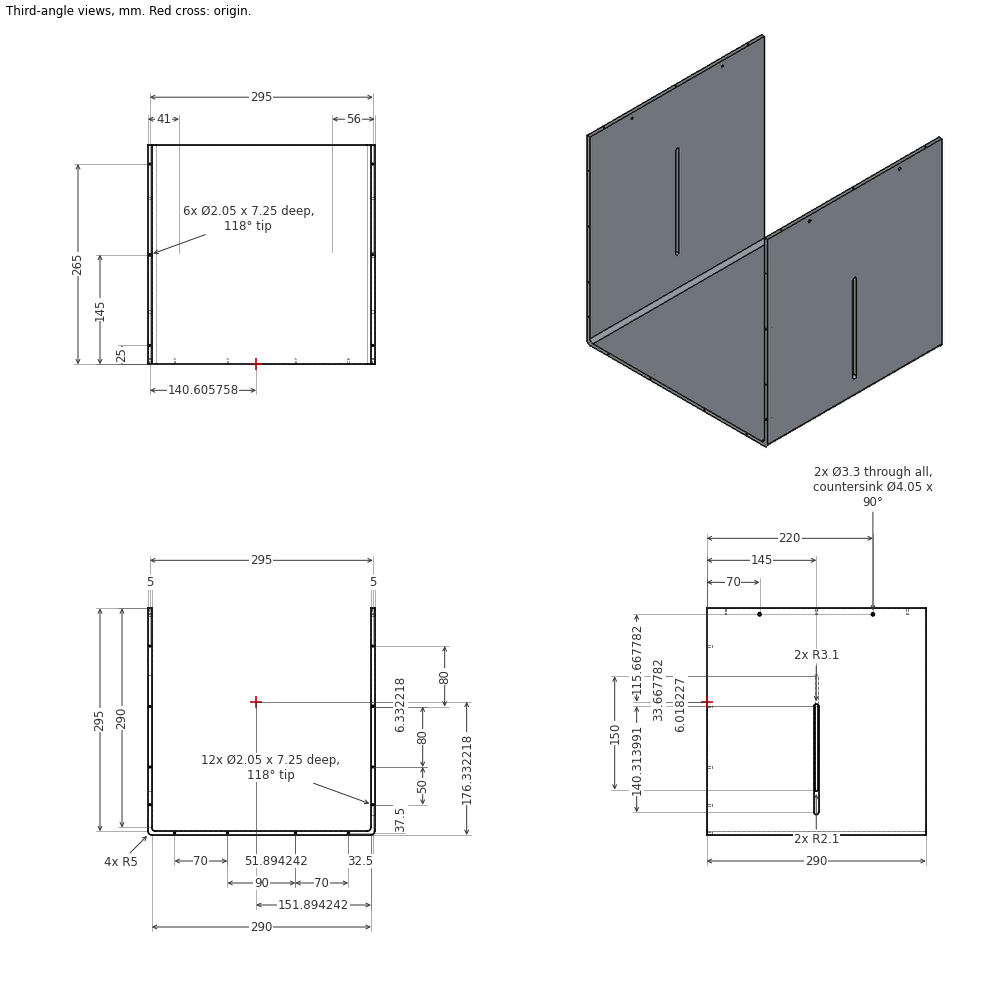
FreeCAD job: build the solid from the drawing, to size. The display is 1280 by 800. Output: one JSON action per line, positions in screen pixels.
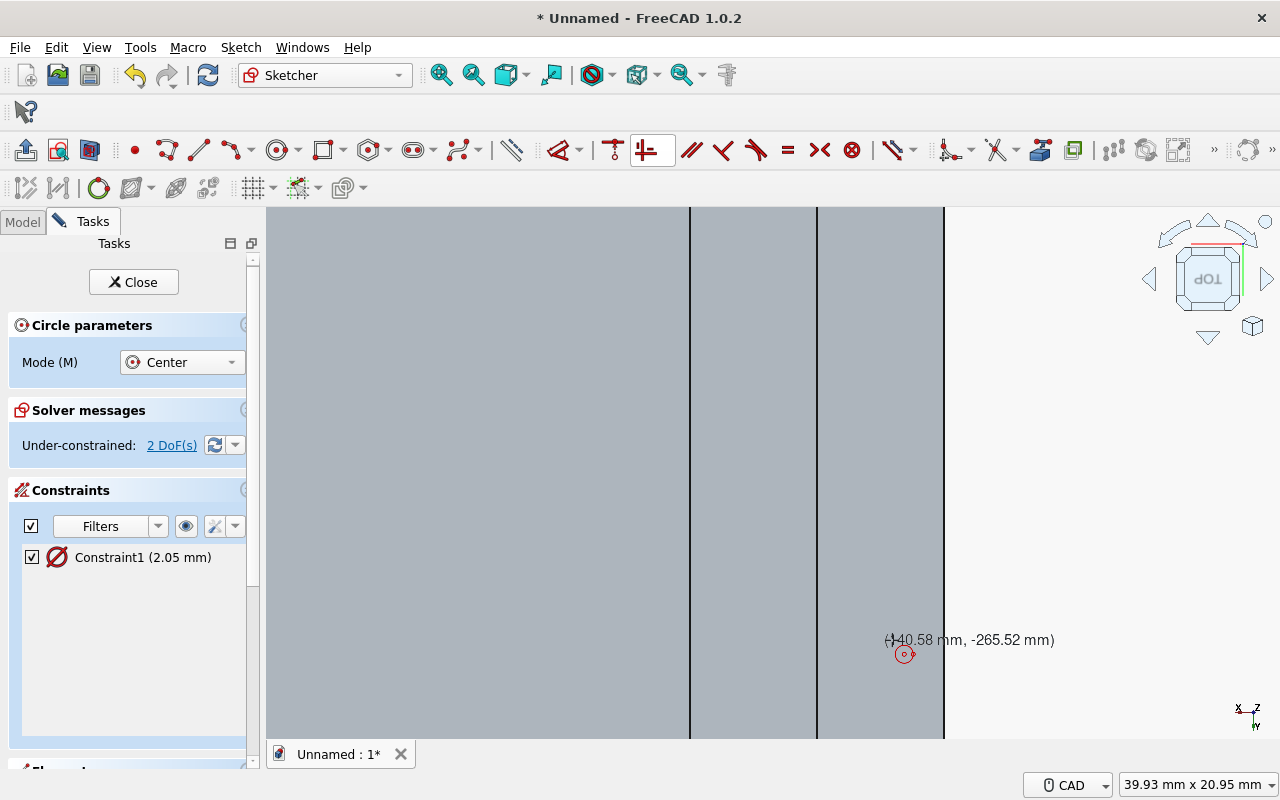
{"action": "scroll", "coordinate": [892, 640], "scroll_direction": "down", "scroll_amount": 15}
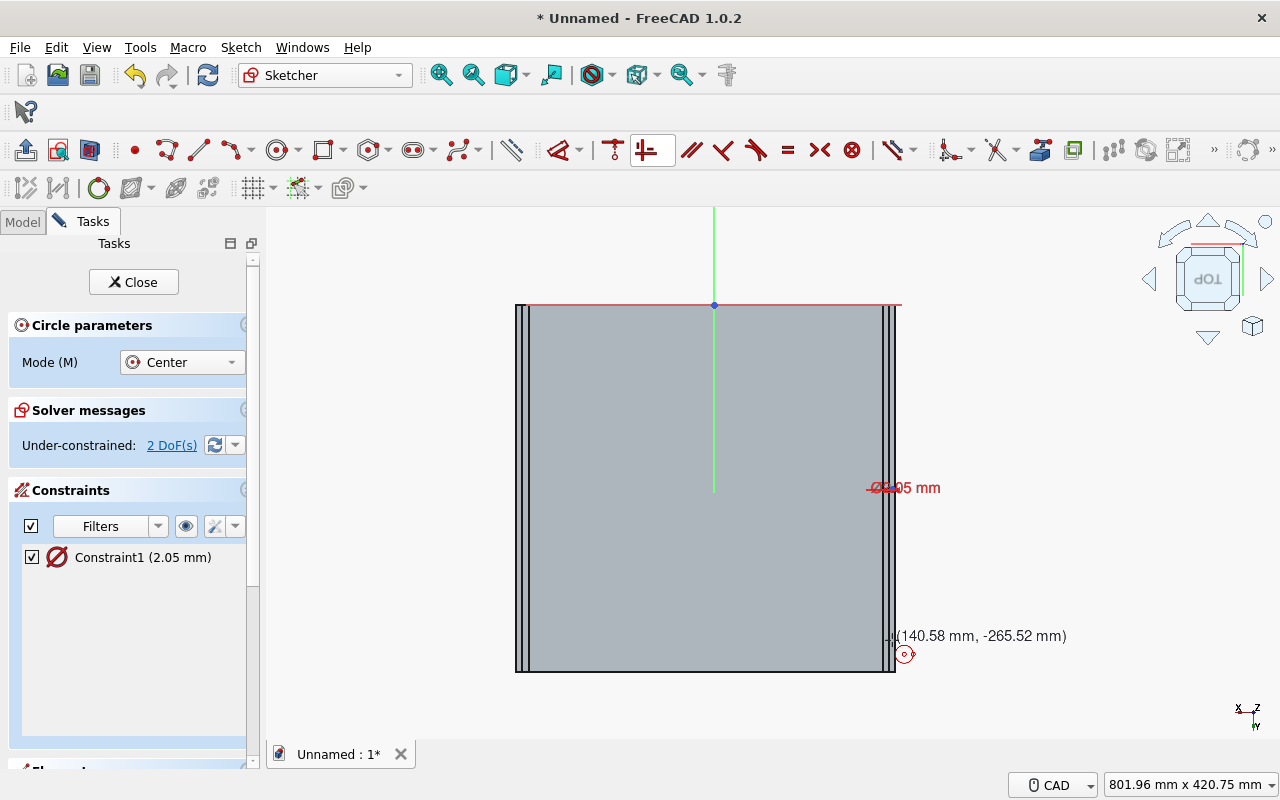
{"action": "left_click", "coordinate": [892, 640]}
{"action": "mouse_move", "coordinate": [893, 639]}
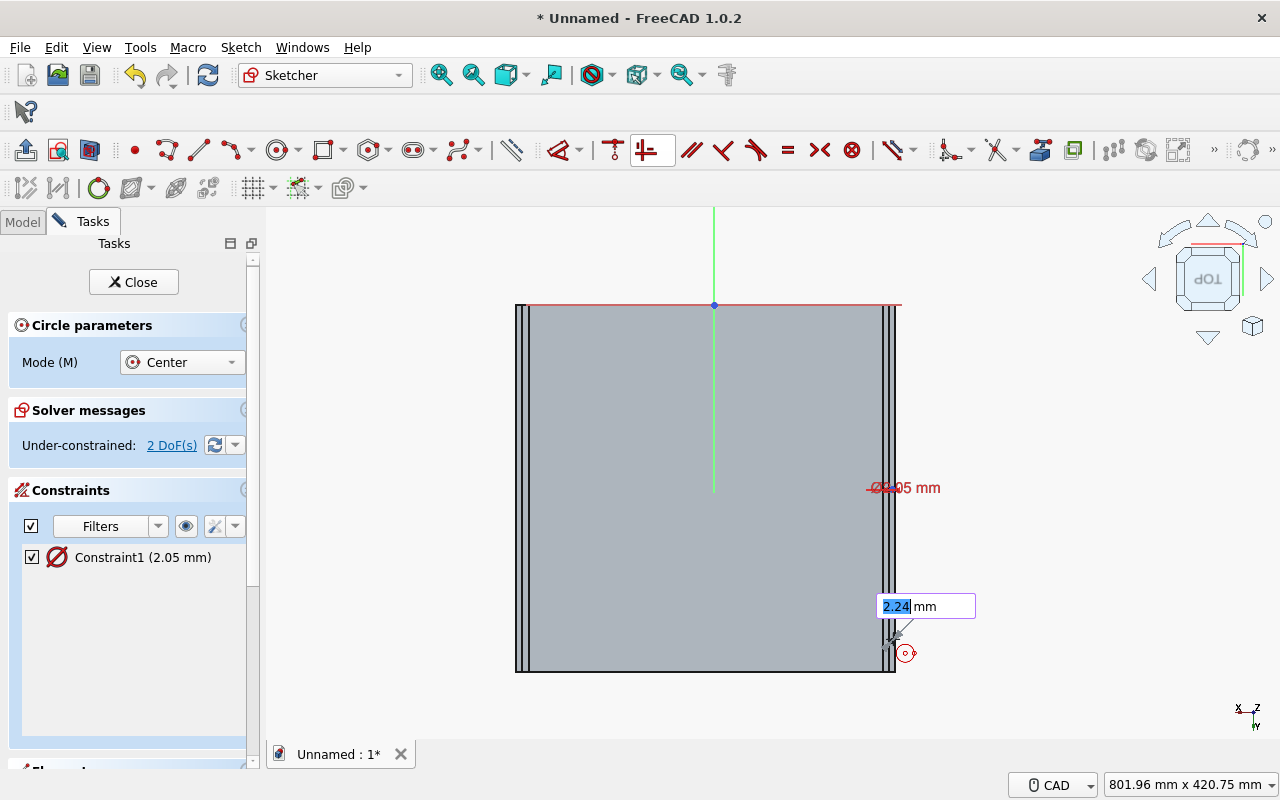
{"action": "type", "text": "2.05"}
{"action": "key", "text": "Return"}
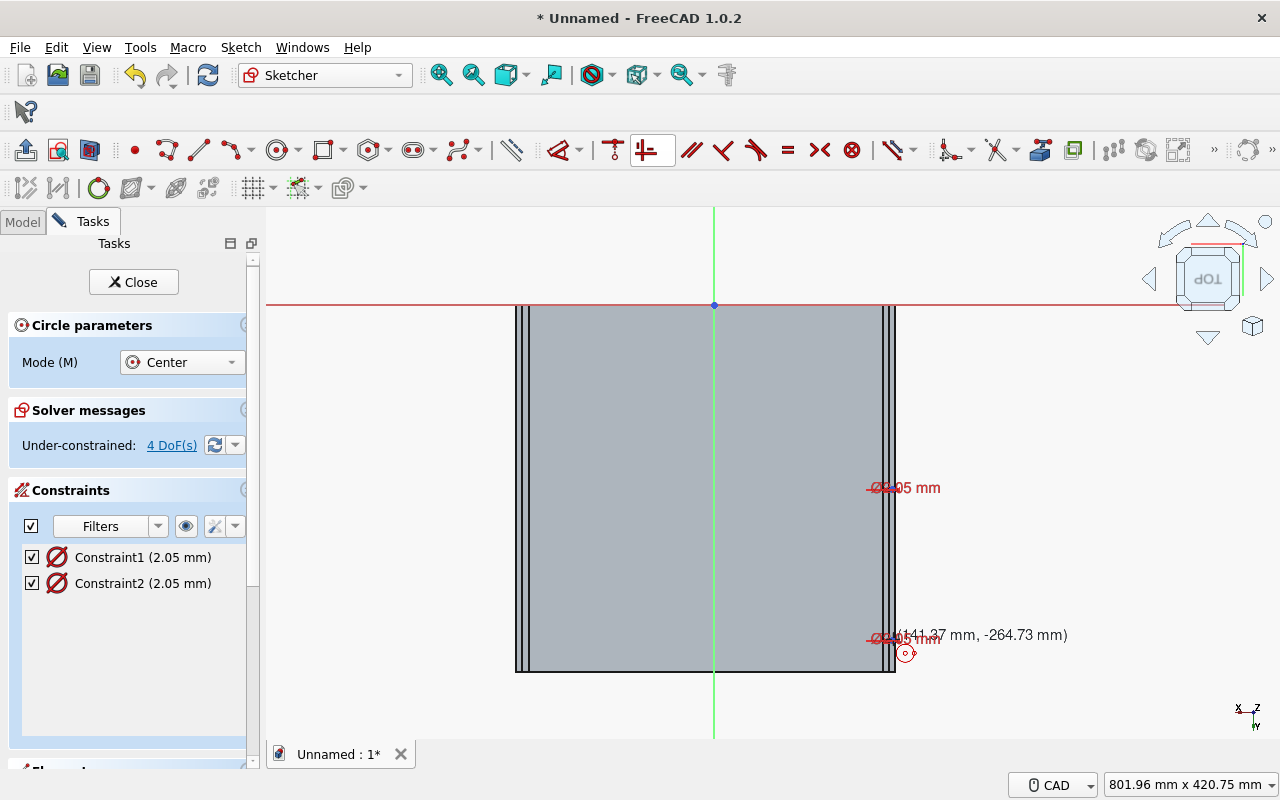
{"action": "scroll", "coordinate": [892, 337], "scroll_direction": "up", "scroll_amount": 15}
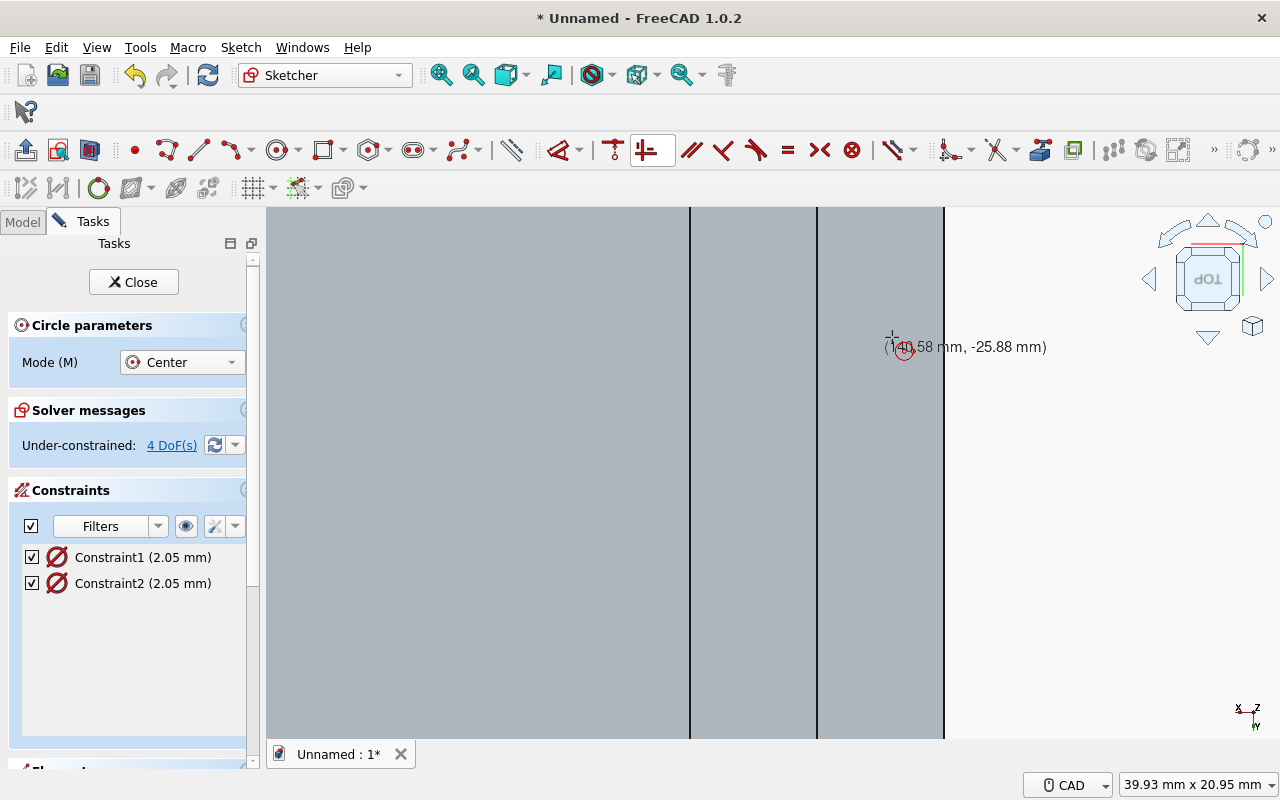
{"action": "scroll", "coordinate": [892, 337], "scroll_direction": "down", "scroll_amount": 15}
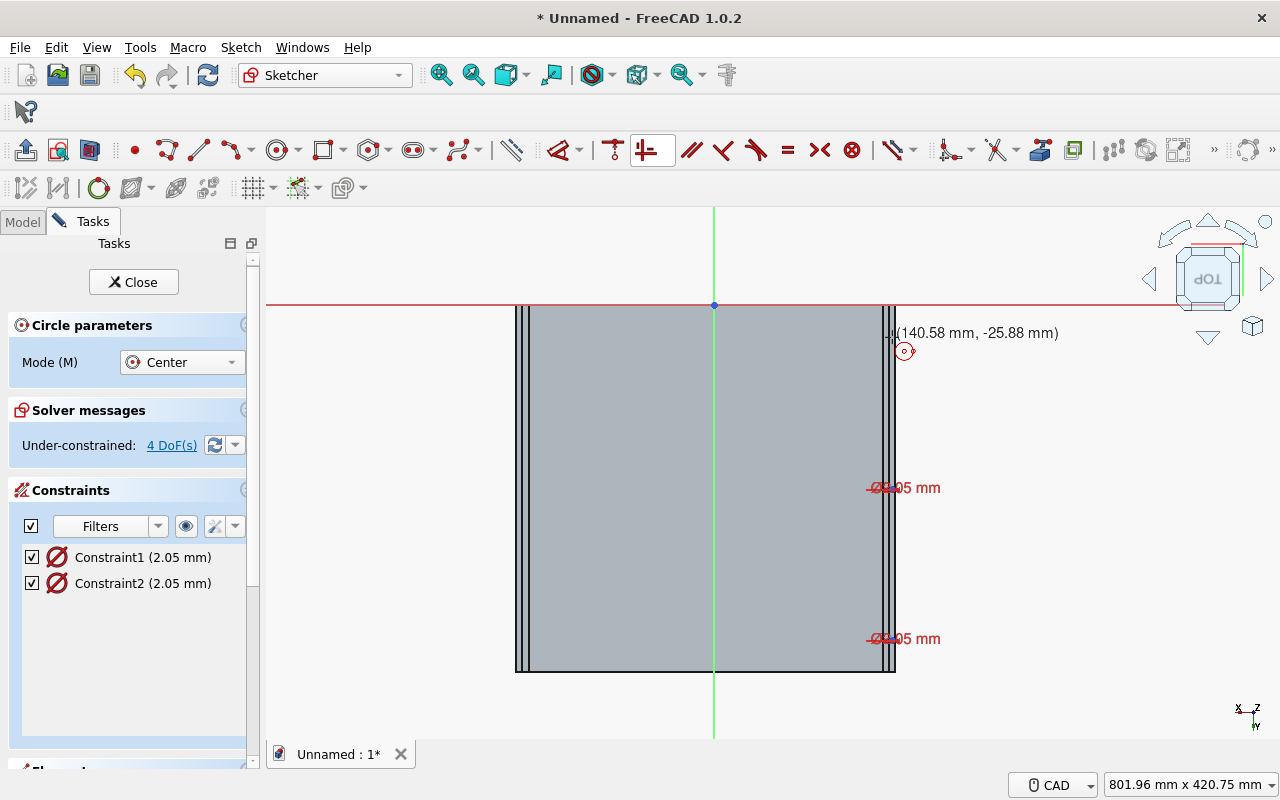
{"action": "left_click", "coordinate": [892, 337]}
{"action": "mouse_move", "coordinate": [893, 336]}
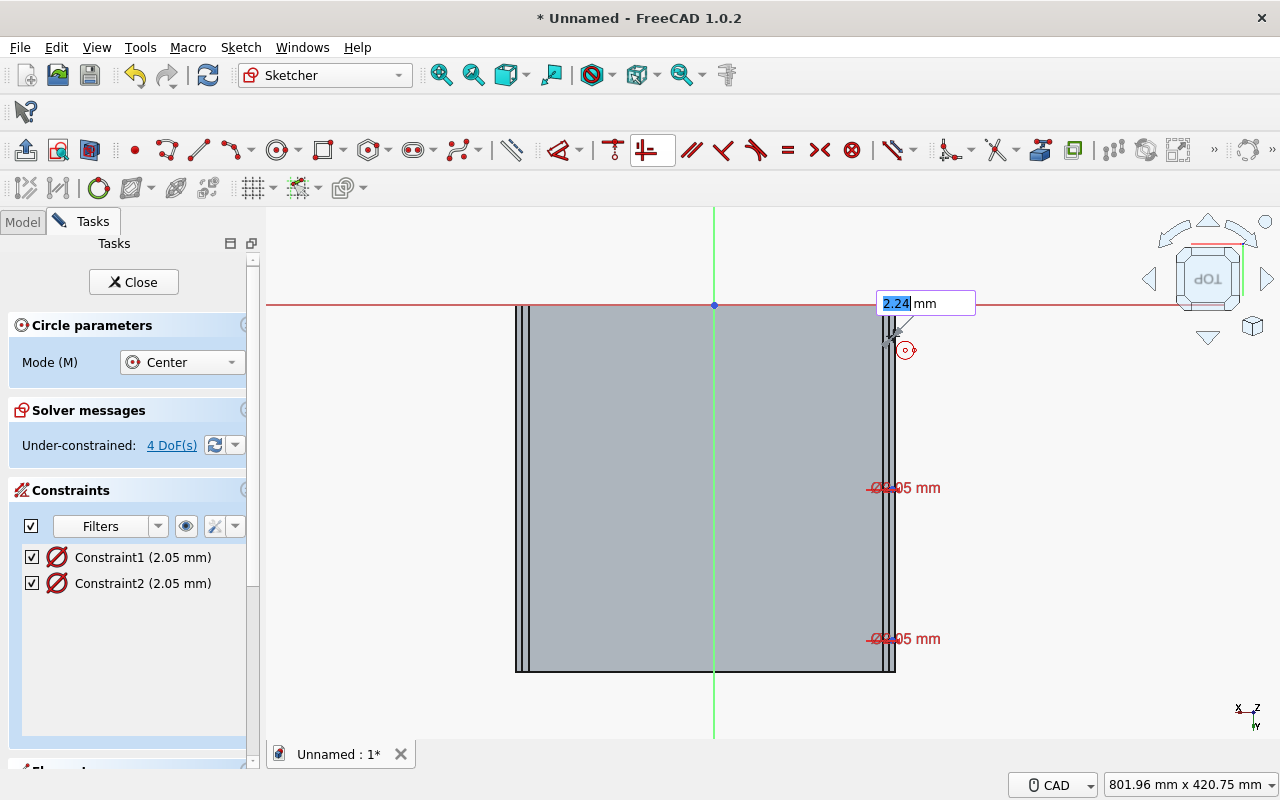
{"action": "type", "text": "2.05"}
{"action": "key", "text": "Return"}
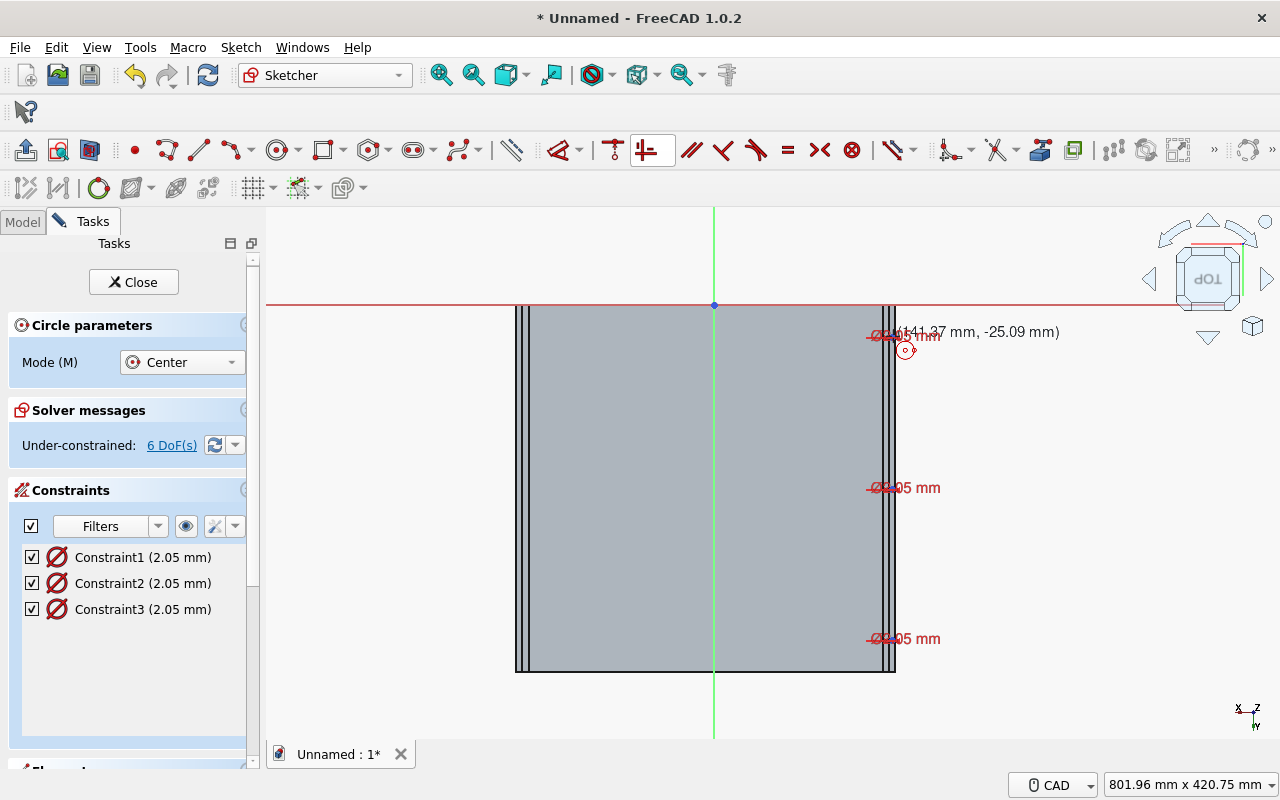
{"action": "scroll", "coordinate": [519, 489], "scroll_direction": "up", "scroll_amount": 15}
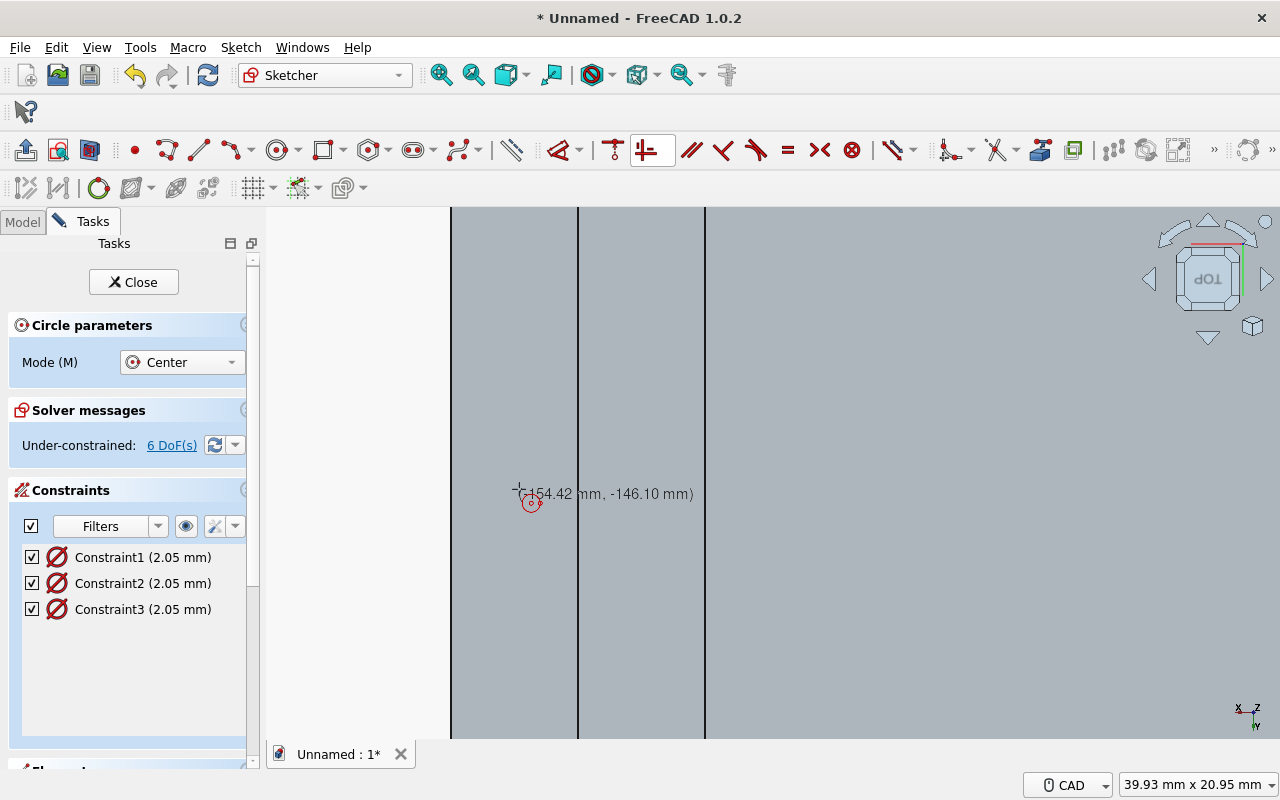
{"action": "scroll", "coordinate": [518, 489], "scroll_direction": "down", "scroll_amount": 15}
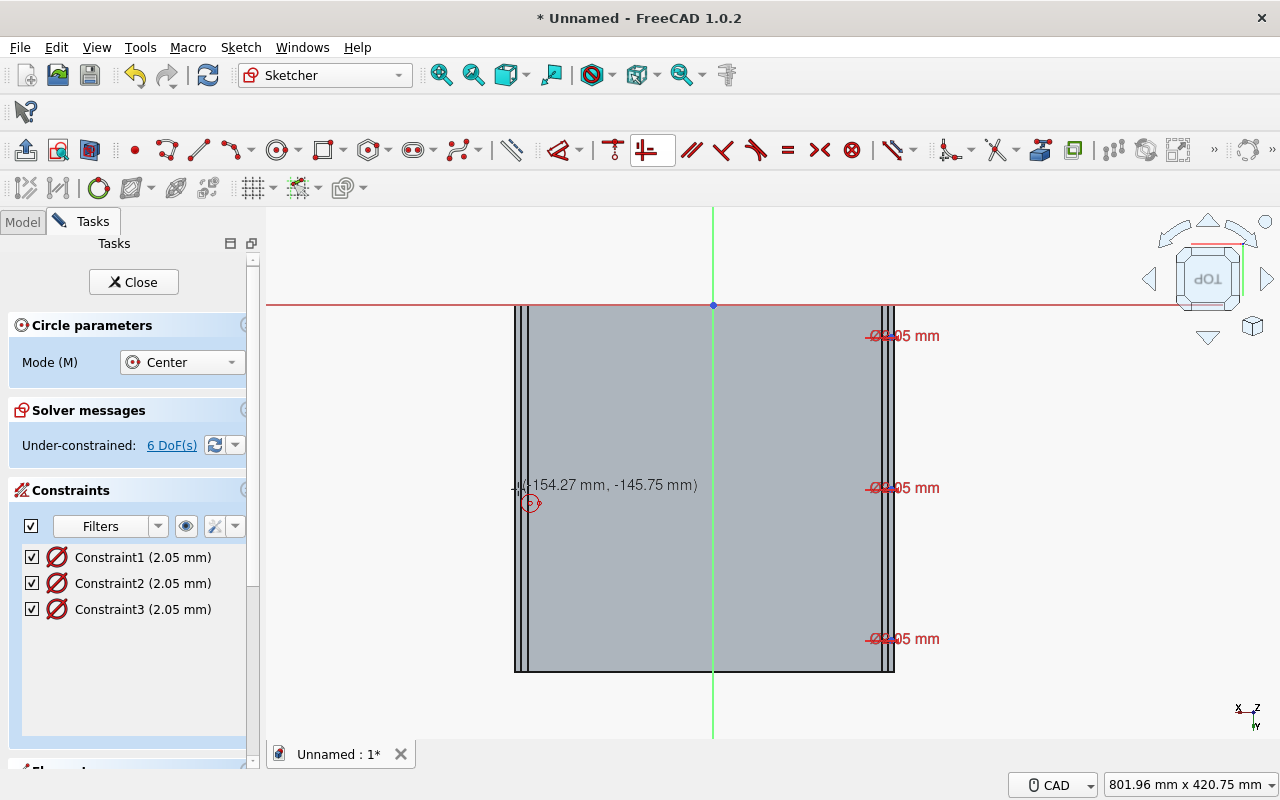
{"action": "left_click", "coordinate": [518, 489]}
{"action": "mouse_move", "coordinate": [519, 488]}